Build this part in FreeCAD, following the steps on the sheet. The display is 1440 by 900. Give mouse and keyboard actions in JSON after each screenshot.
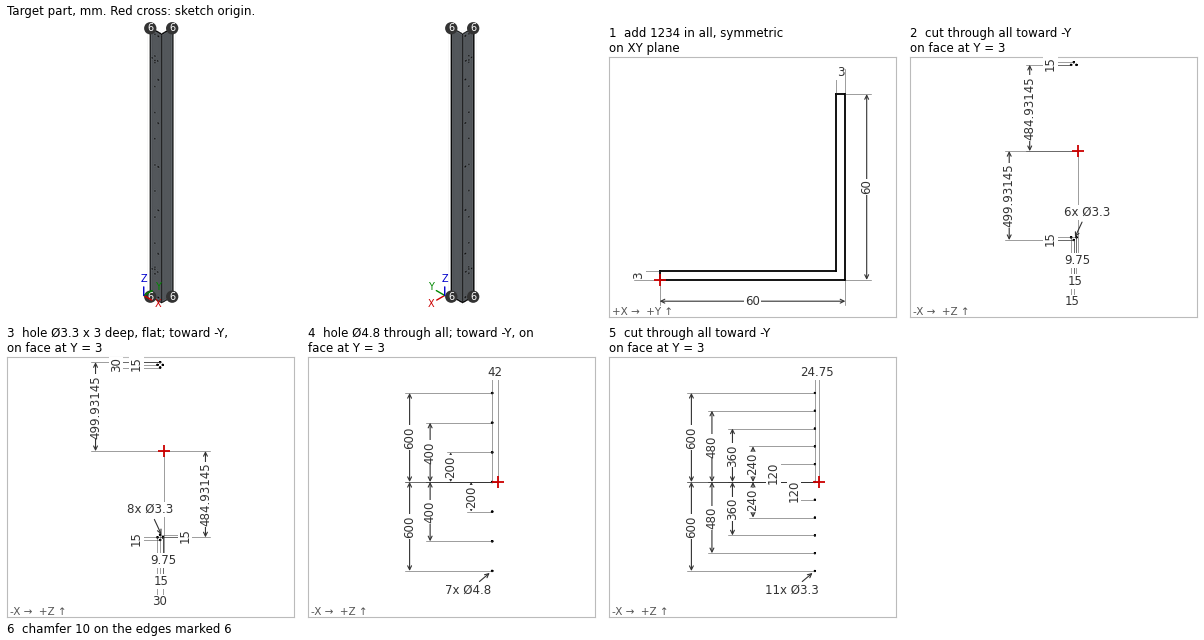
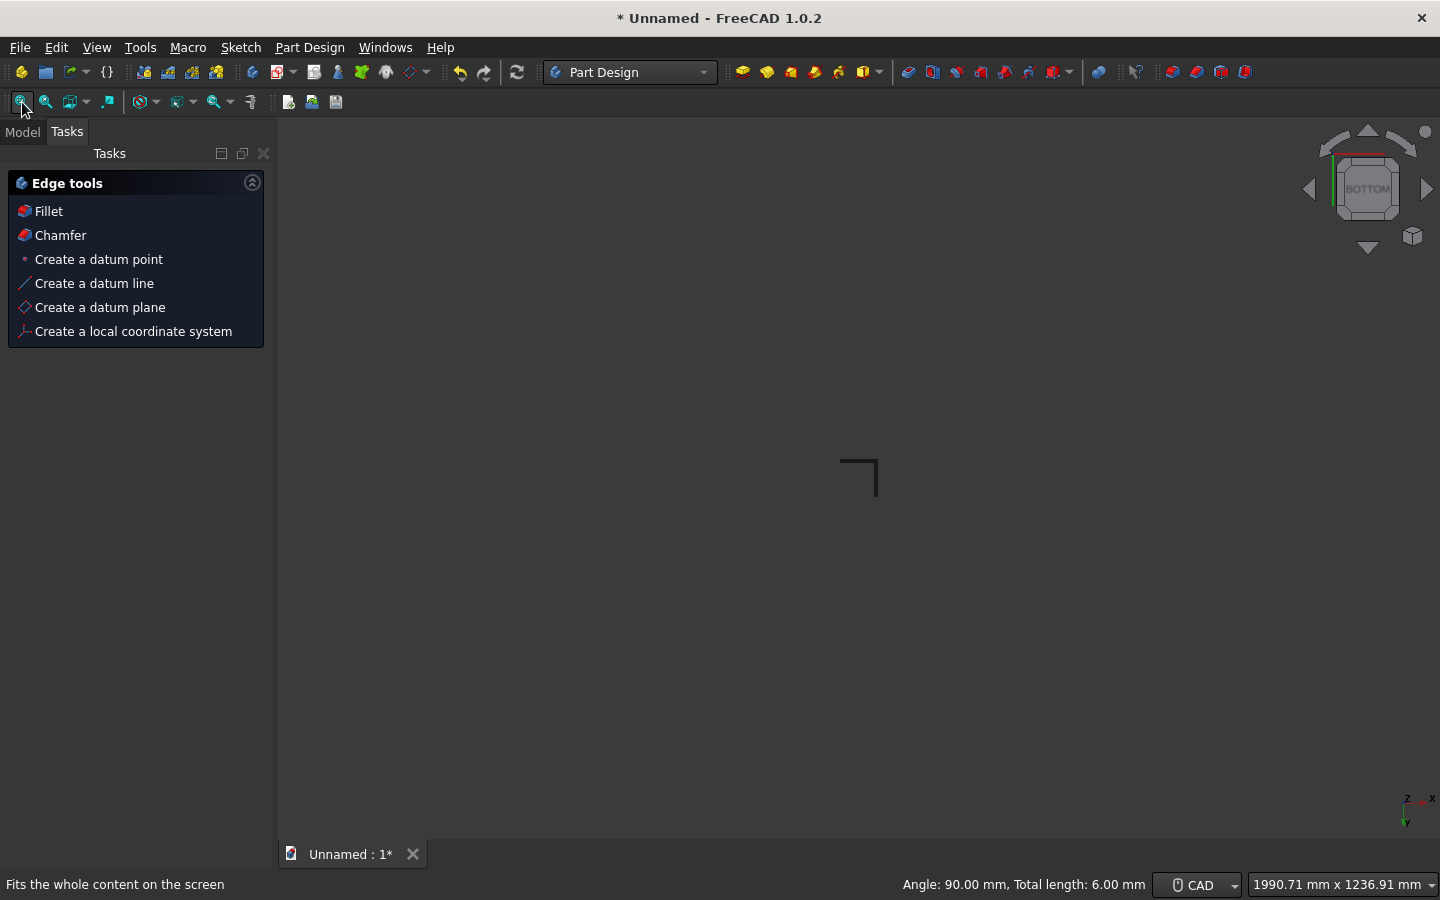
{"action": "key", "text": "4"}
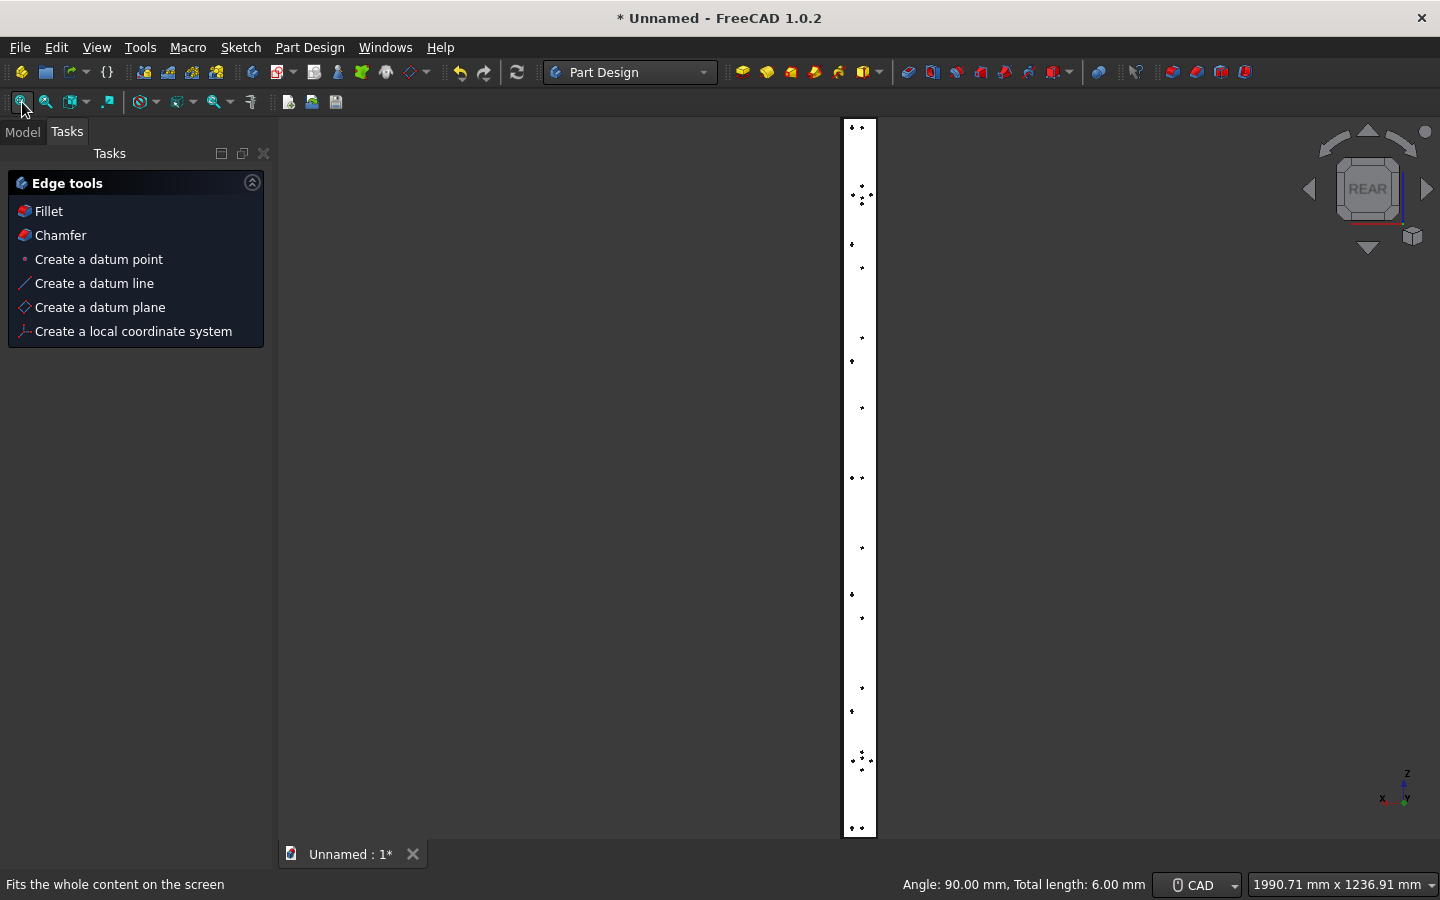
{"action": "key", "text": "6"}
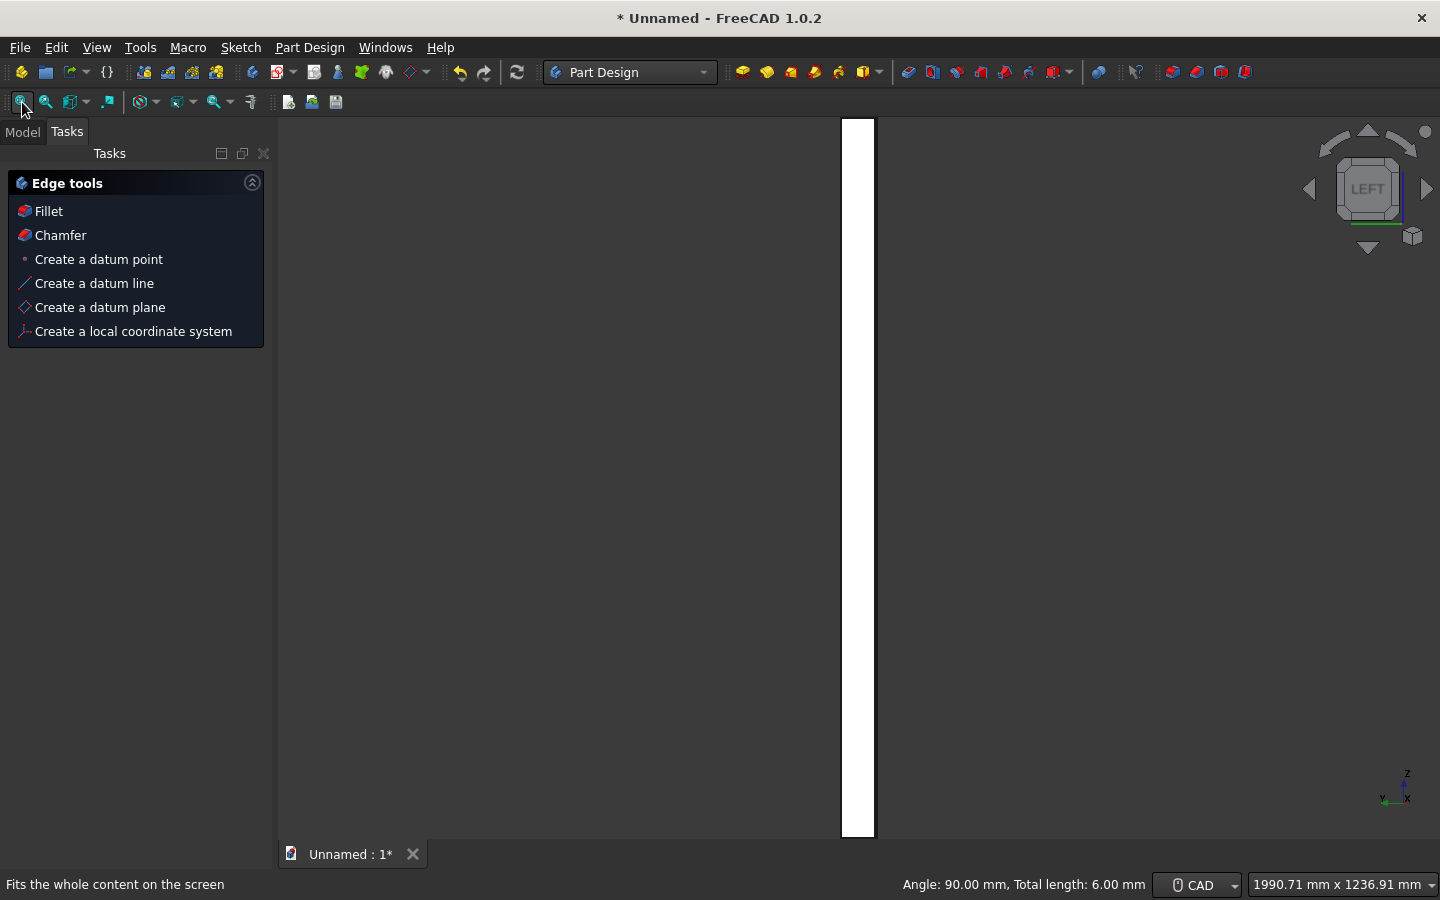
{"action": "key", "text": "v 3"}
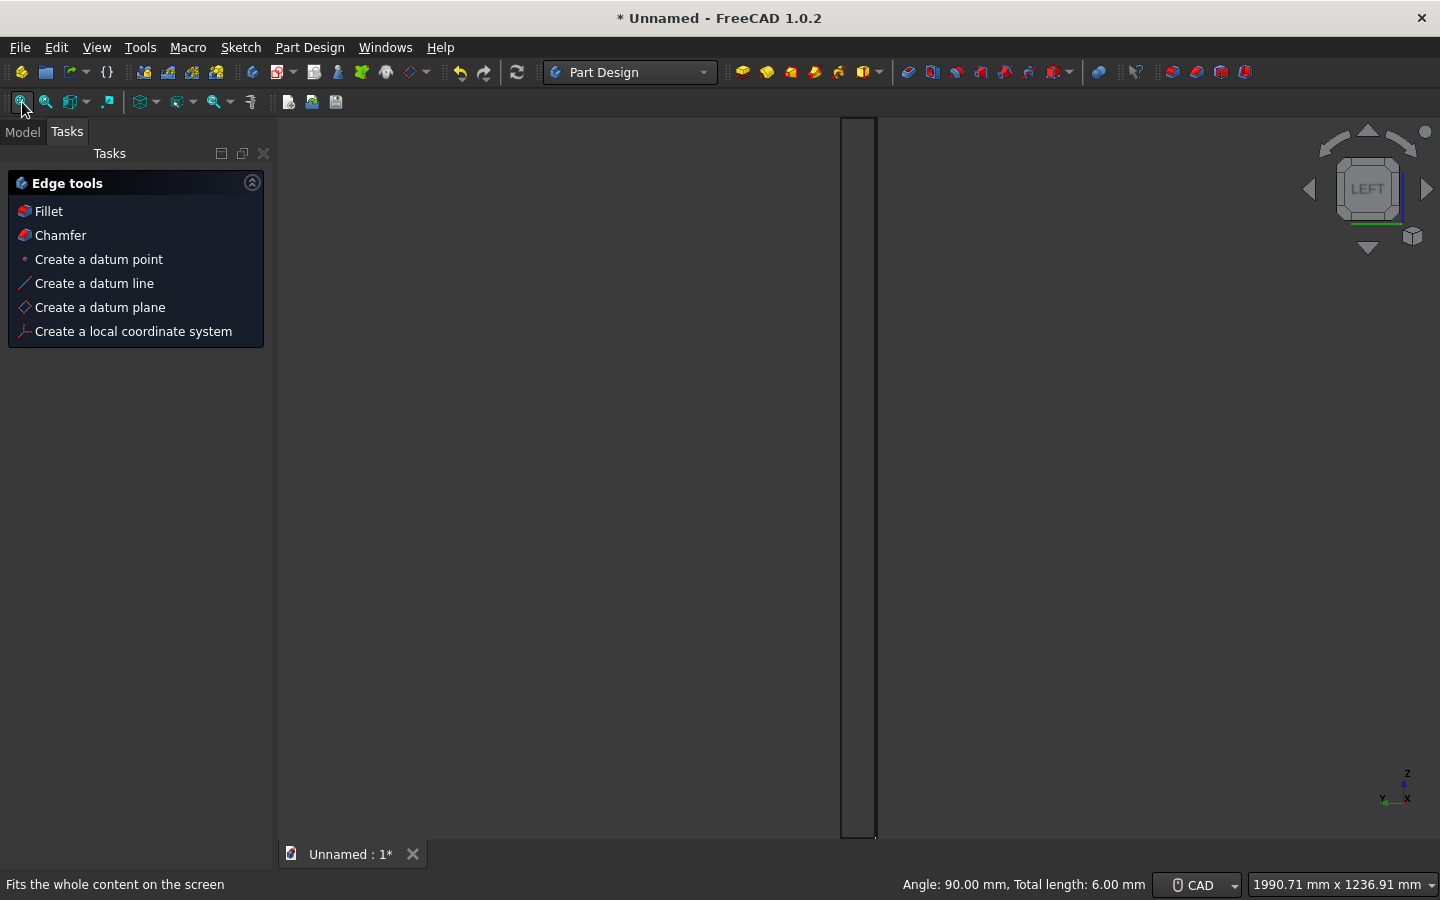
{"action": "key", "text": "0"}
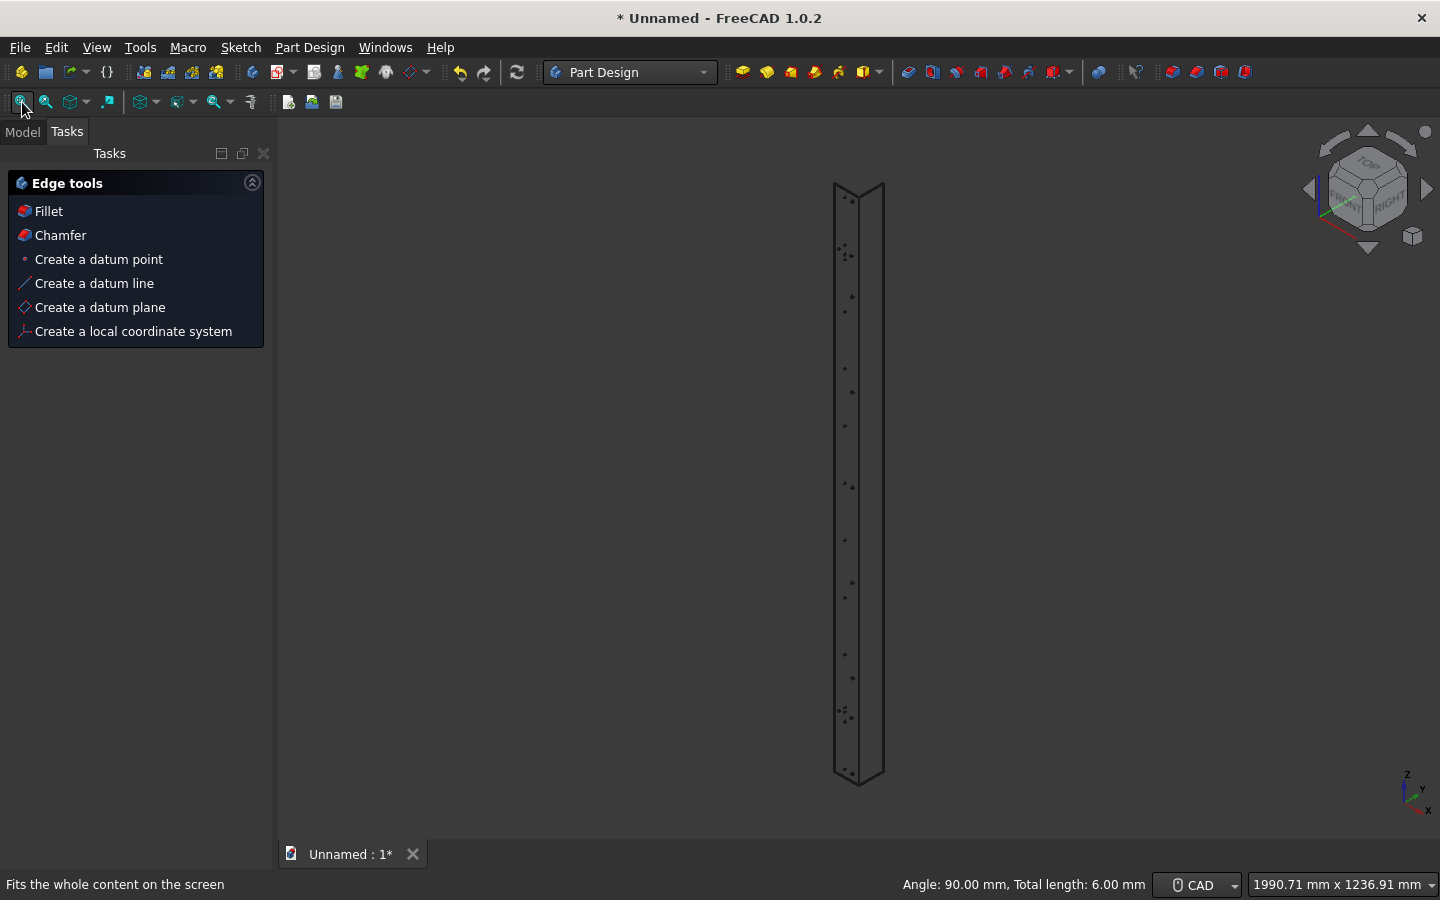
{"action": "scroll", "coordinate": [835, 183], "scroll_direction": "up", "scroll_amount": 15}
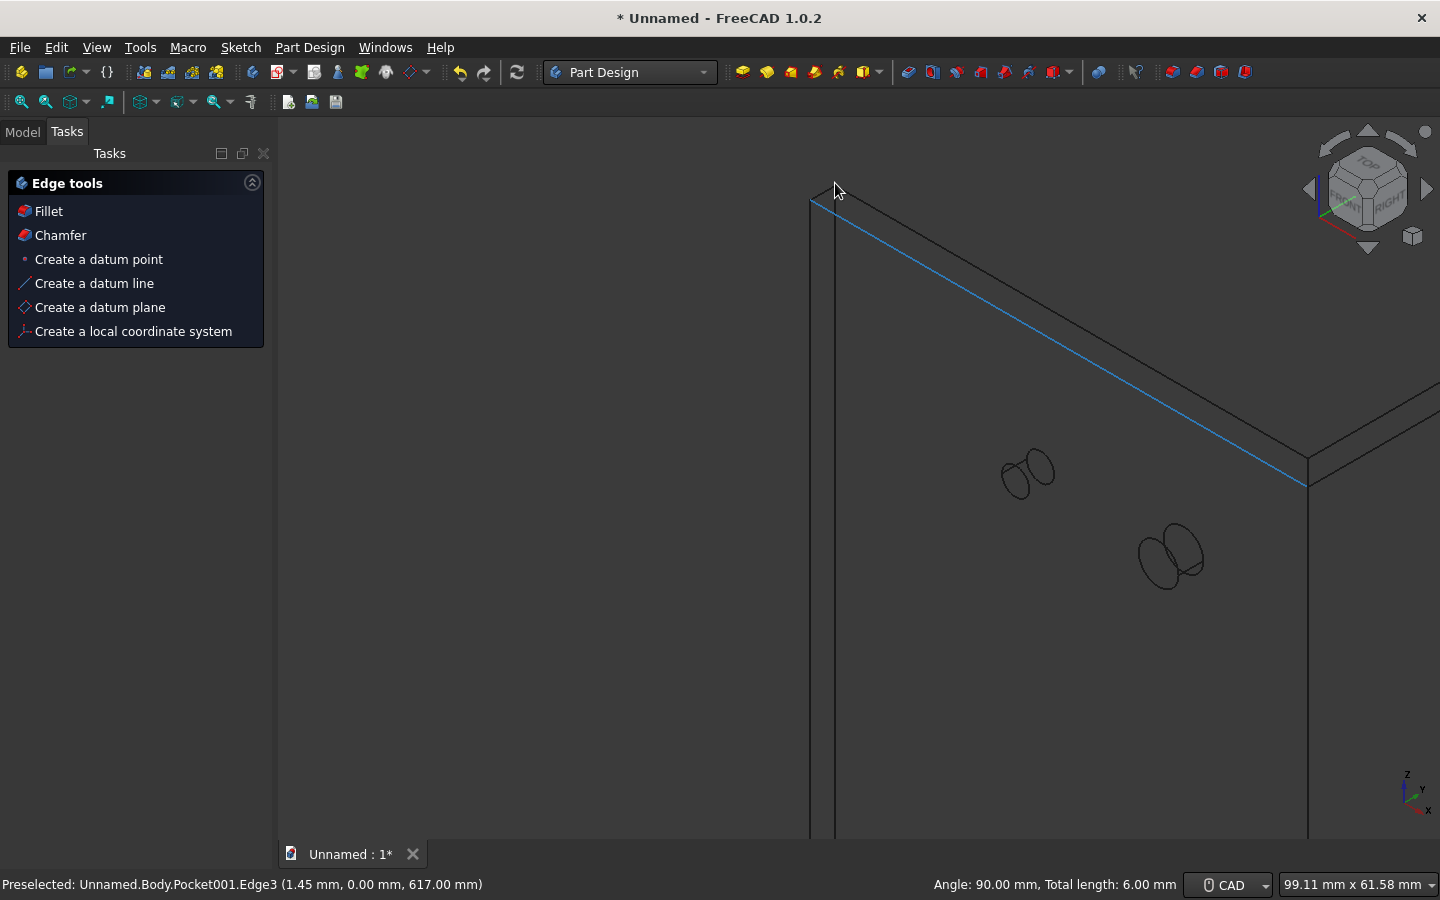
{"action": "left_click", "coordinate": [823, 192], "text": "ctrl"}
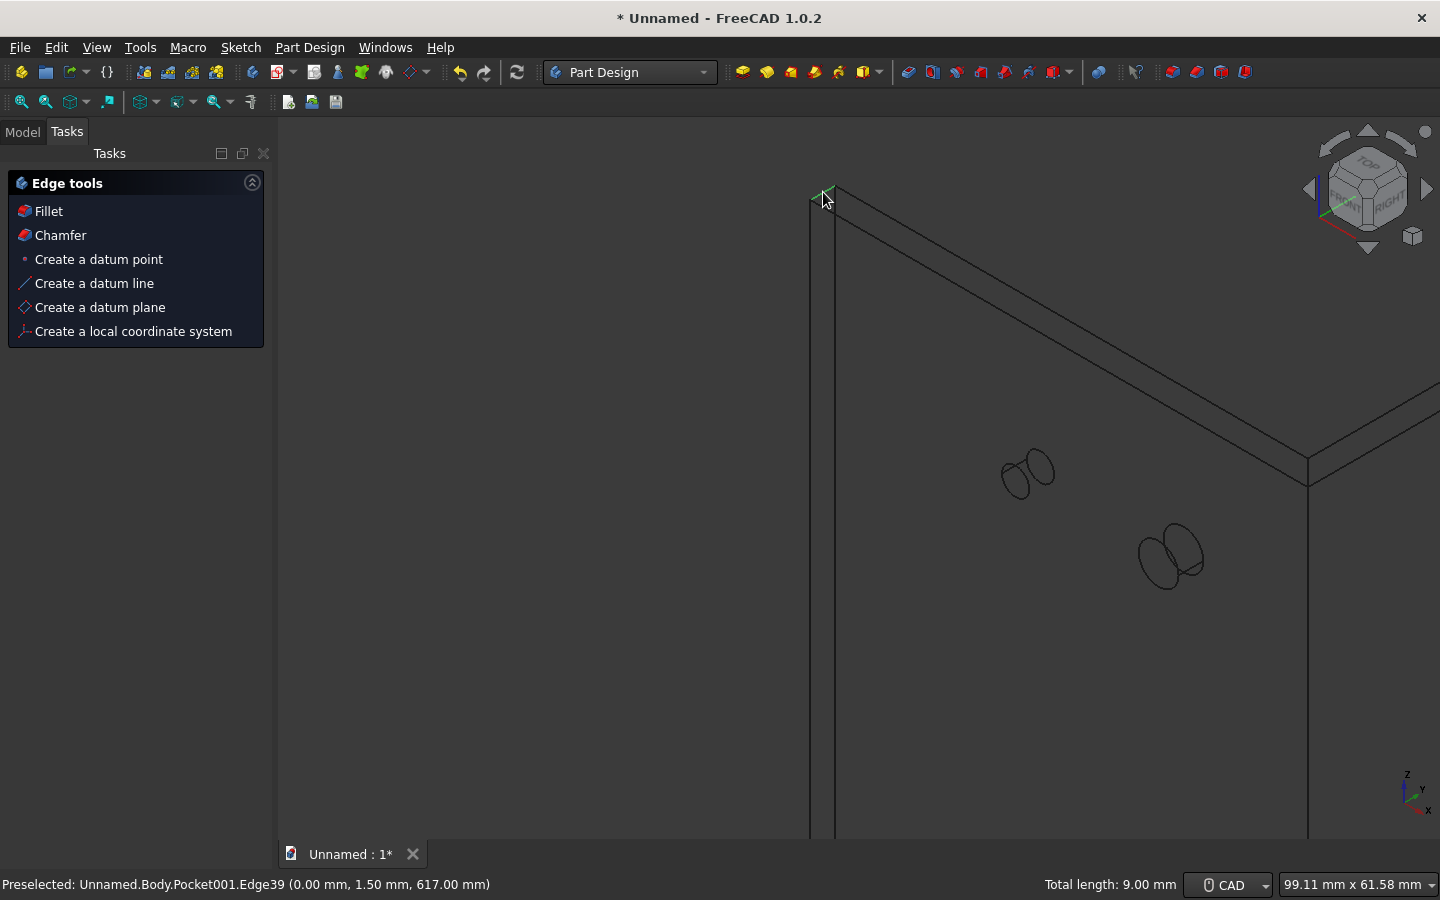
{"action": "left_click", "coordinate": [22, 102]}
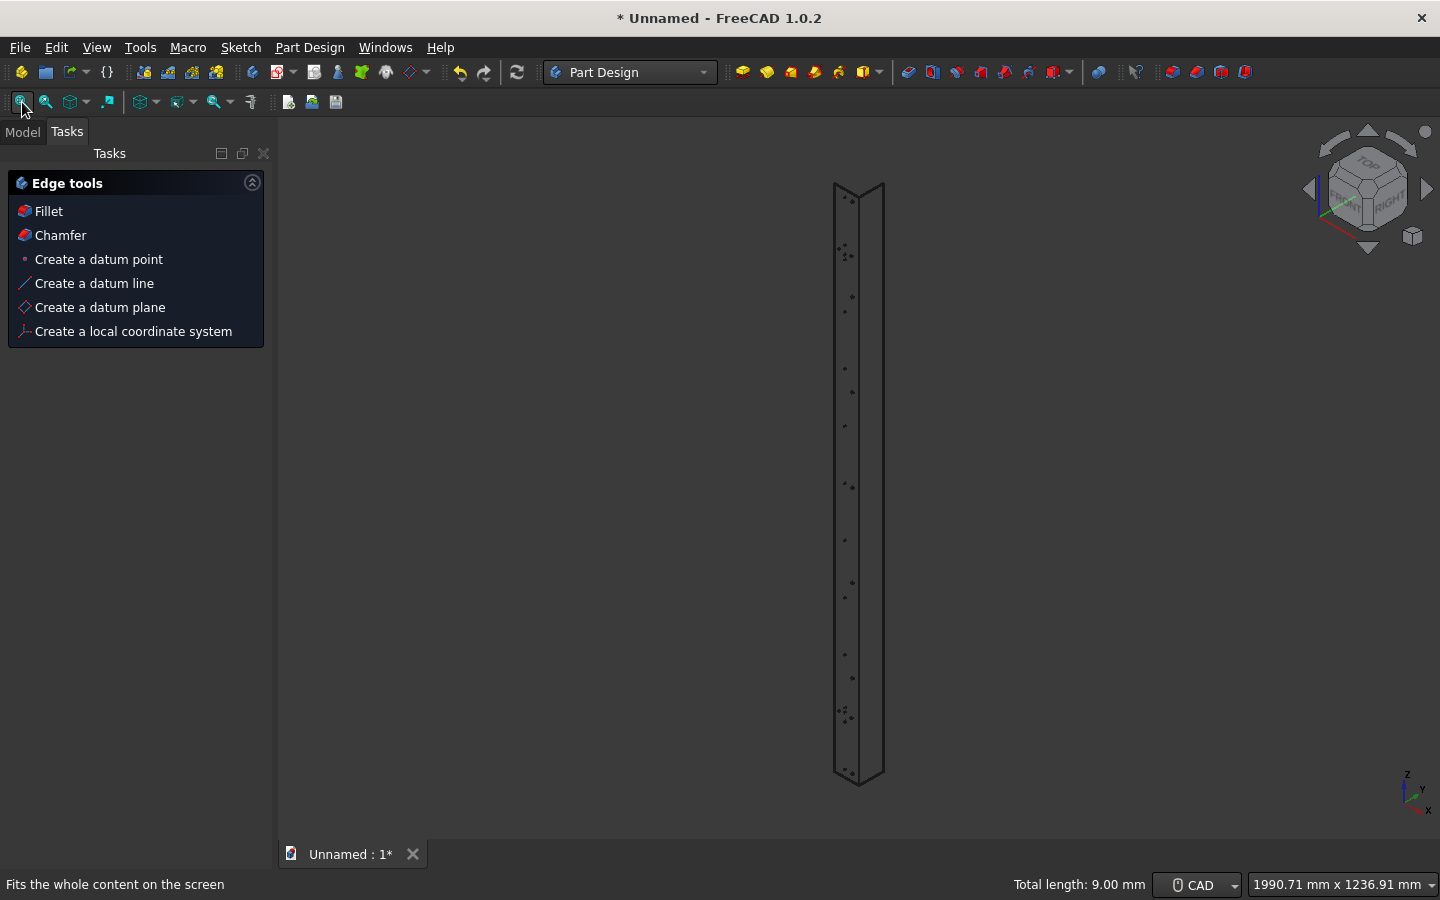
{"action": "key", "text": "2"}